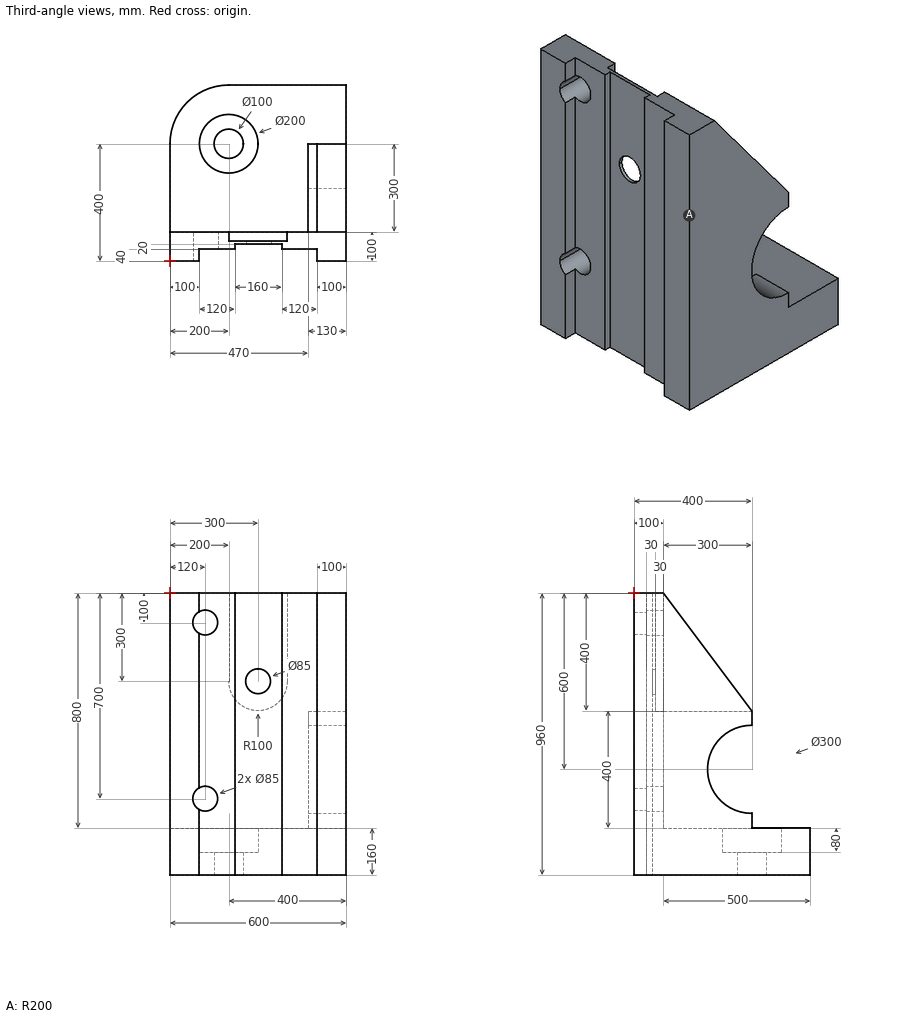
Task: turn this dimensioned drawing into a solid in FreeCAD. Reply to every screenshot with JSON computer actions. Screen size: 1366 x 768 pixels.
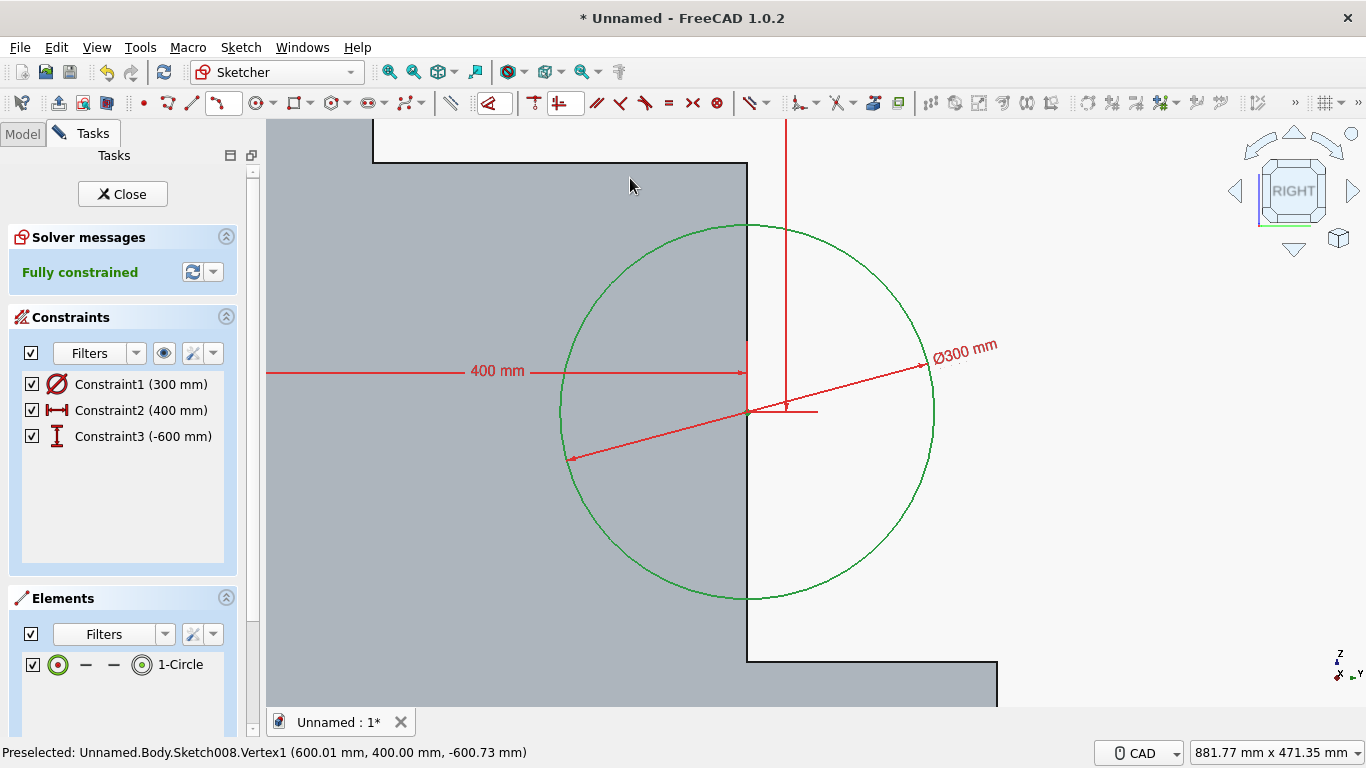
{"action": "left_click", "coordinate": [123, 194]}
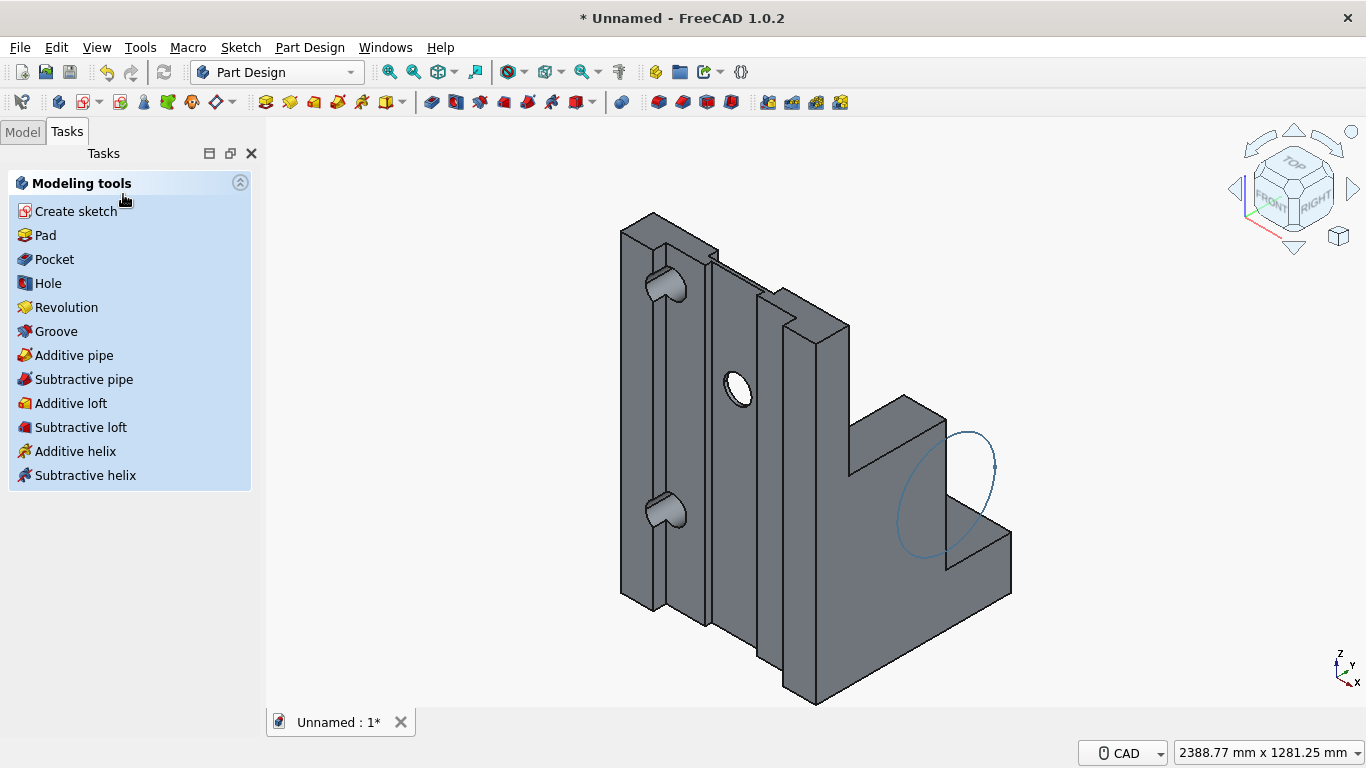
{"action": "left_click", "coordinate": [432, 102]}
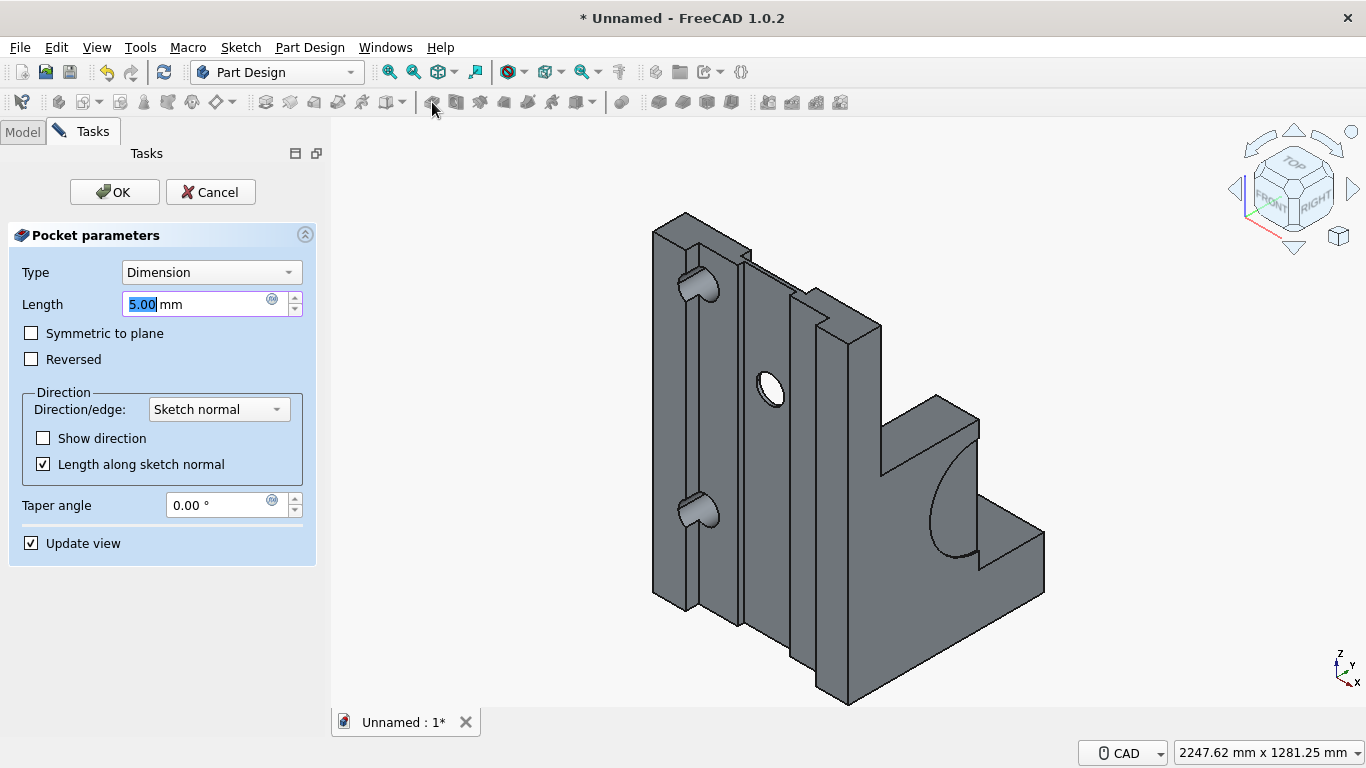
{"action": "type", "text": "400"}
{"action": "key", "text": "Tab"}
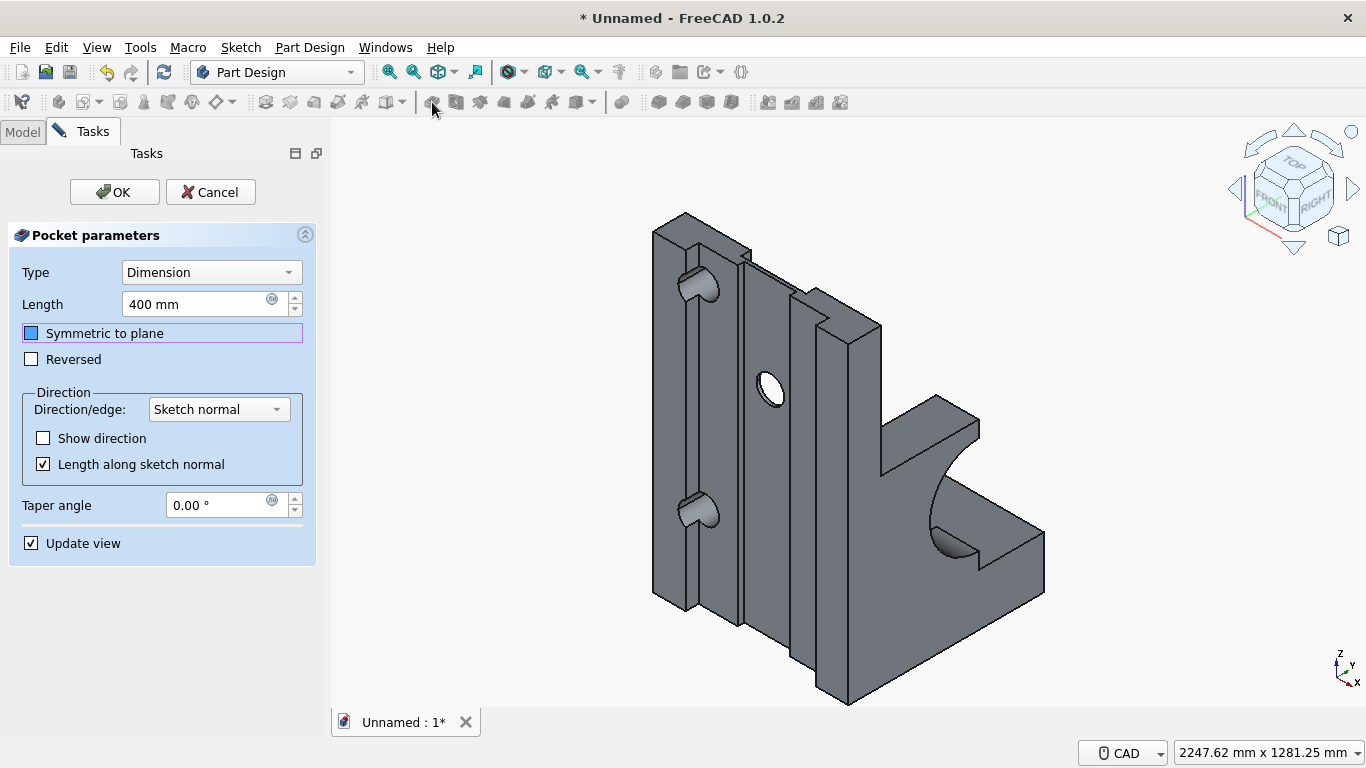
{"action": "left_click", "coordinate": [115, 192]}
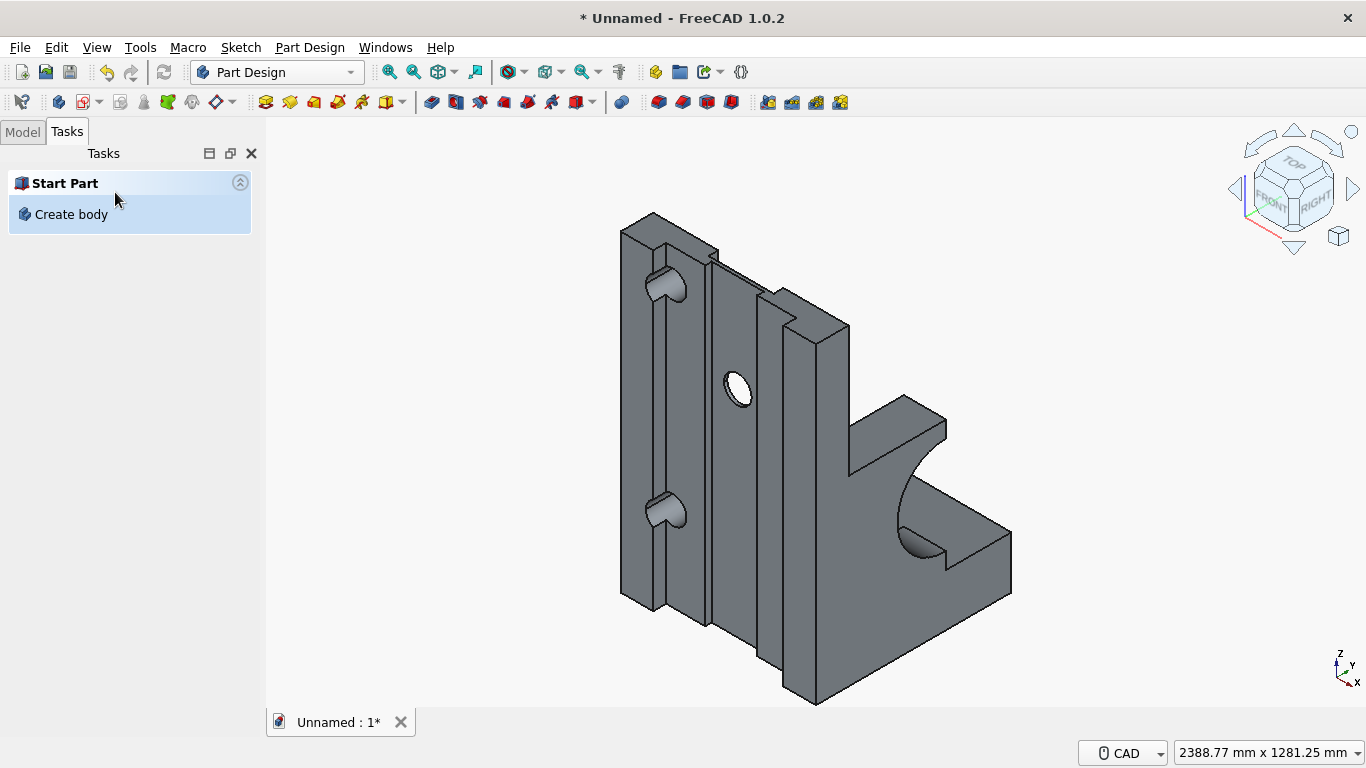
{"action": "left_click", "coordinate": [858, 603]}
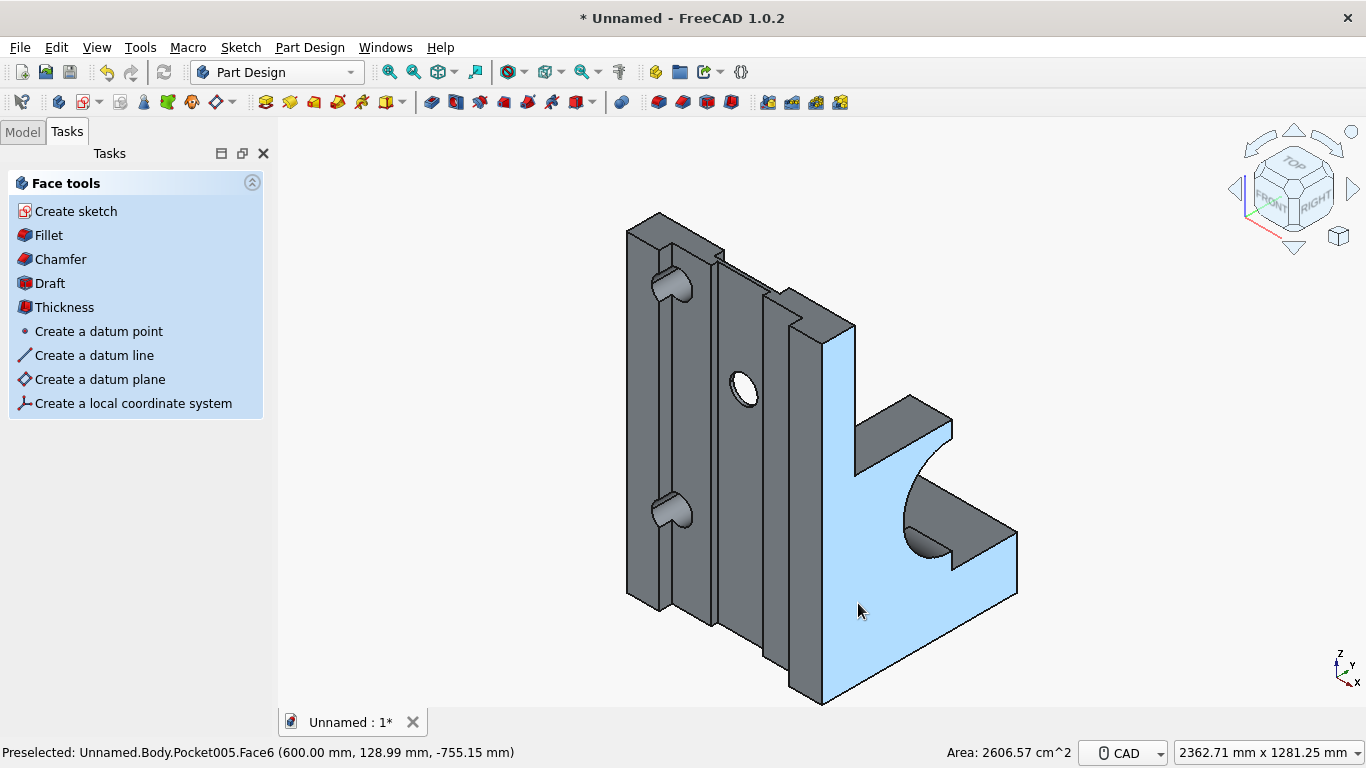
{"action": "left_click", "coordinate": [84, 102]}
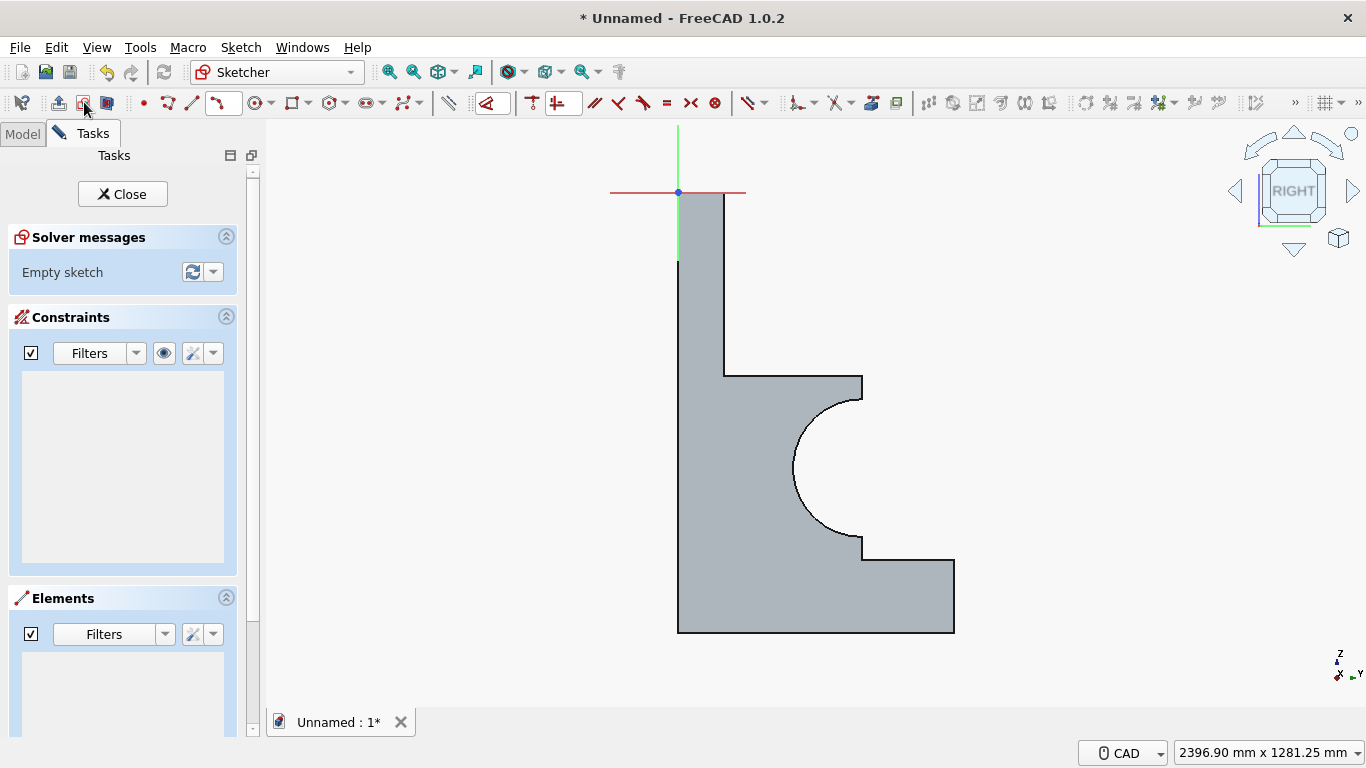
{"action": "scroll", "coordinate": [789, 180], "scroll_direction": "up", "scroll_amount": 4}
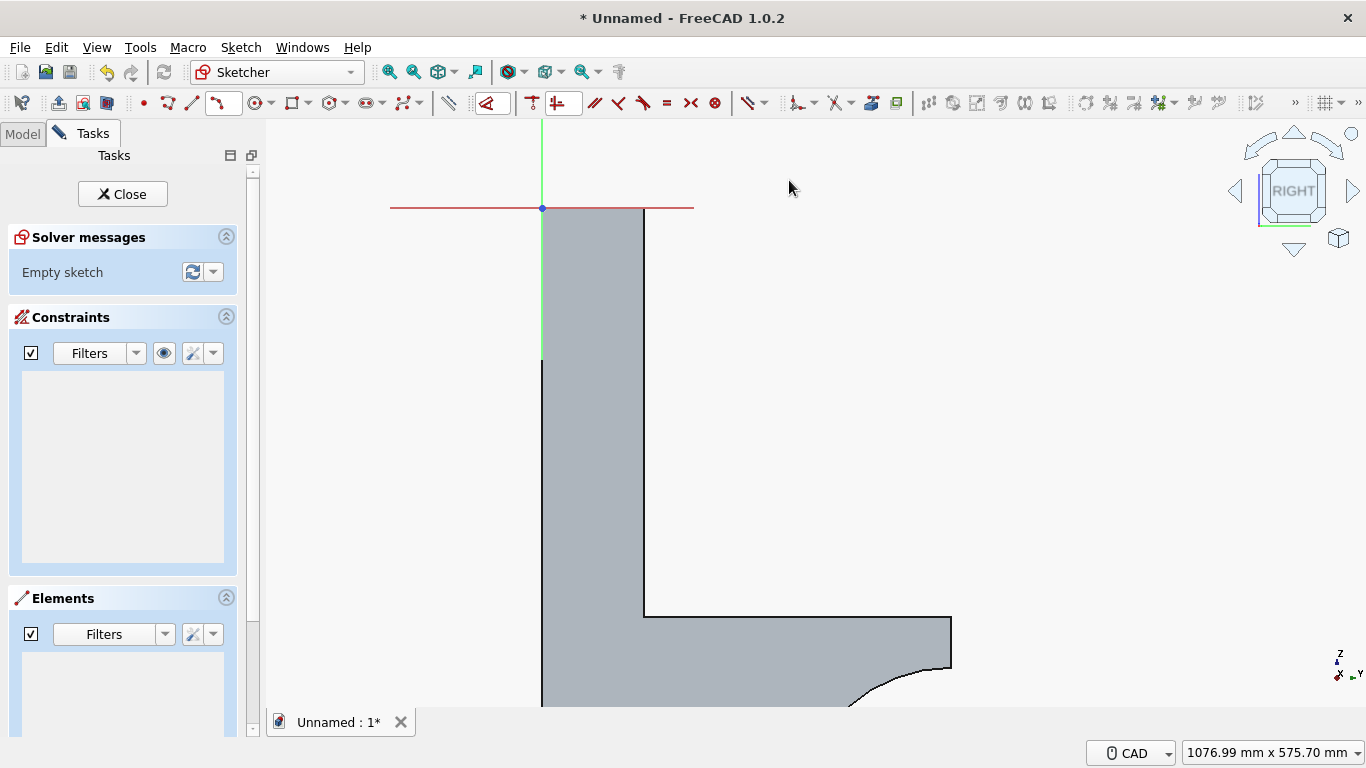
{"action": "left_click", "coordinate": [168, 104]}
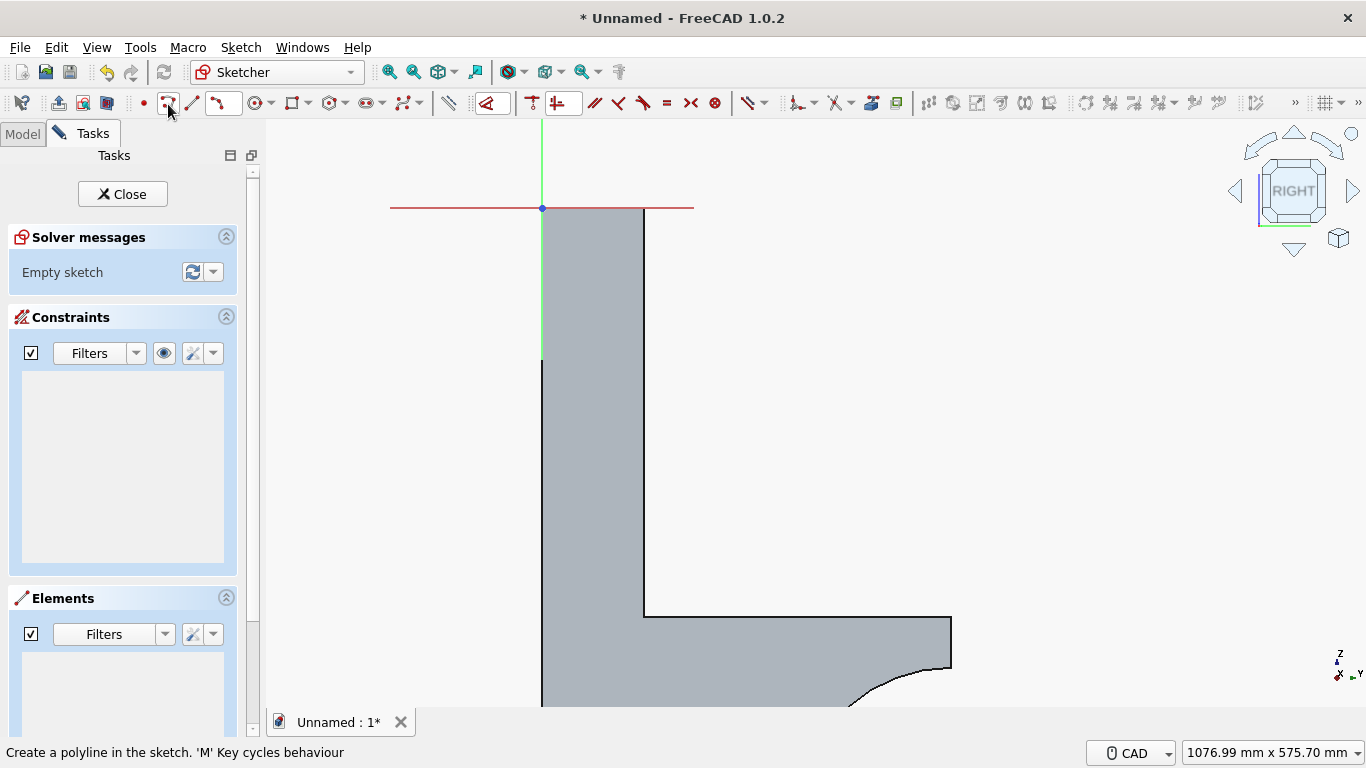
{"action": "left_click", "coordinate": [644, 208]}
{"action": "left_click", "coordinate": [644, 617]}
{"action": "left_click", "coordinate": [951, 617]}
{"action": "left_click", "coordinate": [644, 208]}
{"action": "key", "text": "Escape"}
{"action": "key", "text": "Escape"}